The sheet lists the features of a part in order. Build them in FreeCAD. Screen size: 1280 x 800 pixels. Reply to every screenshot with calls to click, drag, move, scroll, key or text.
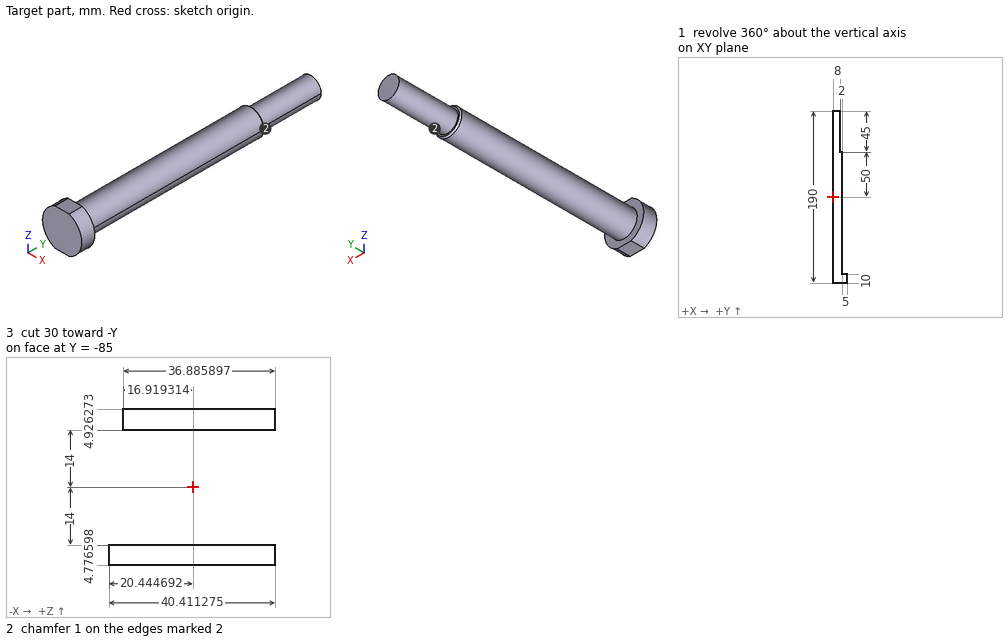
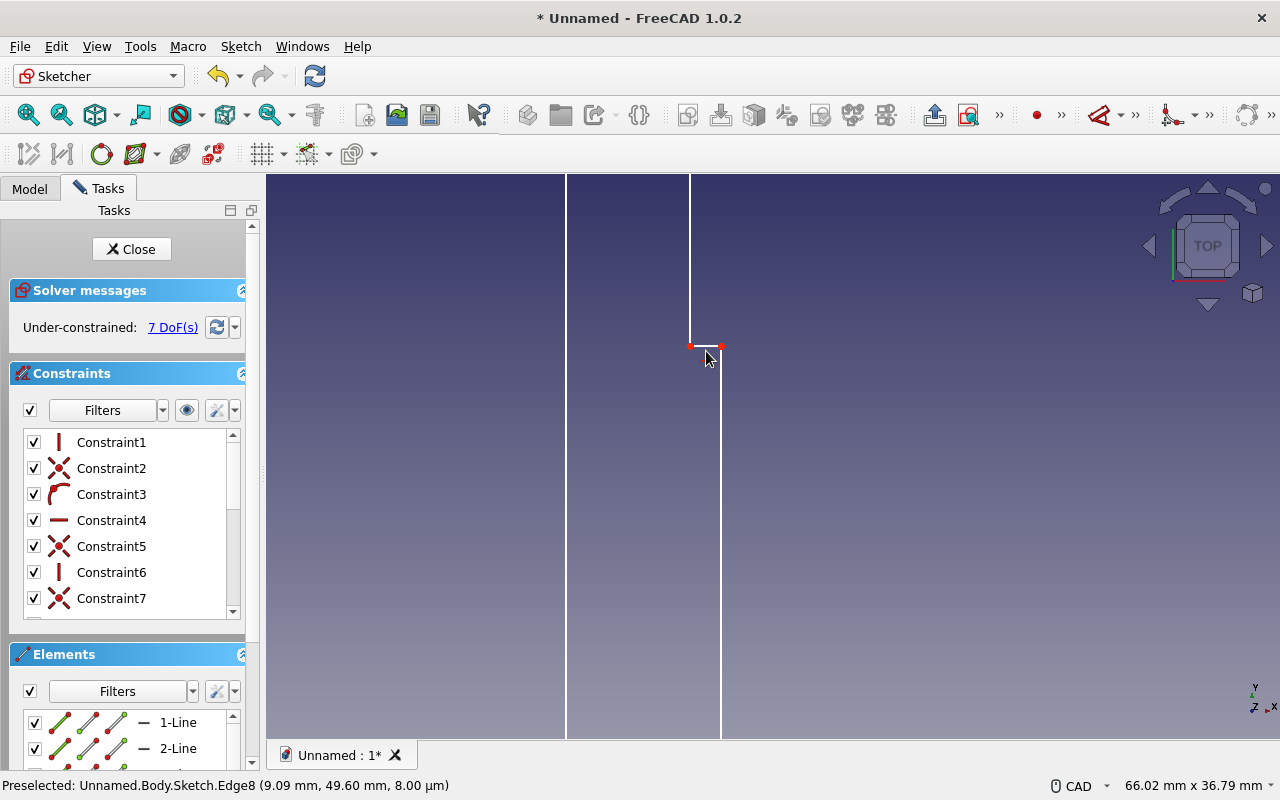
scroll(708, 354, down, 10)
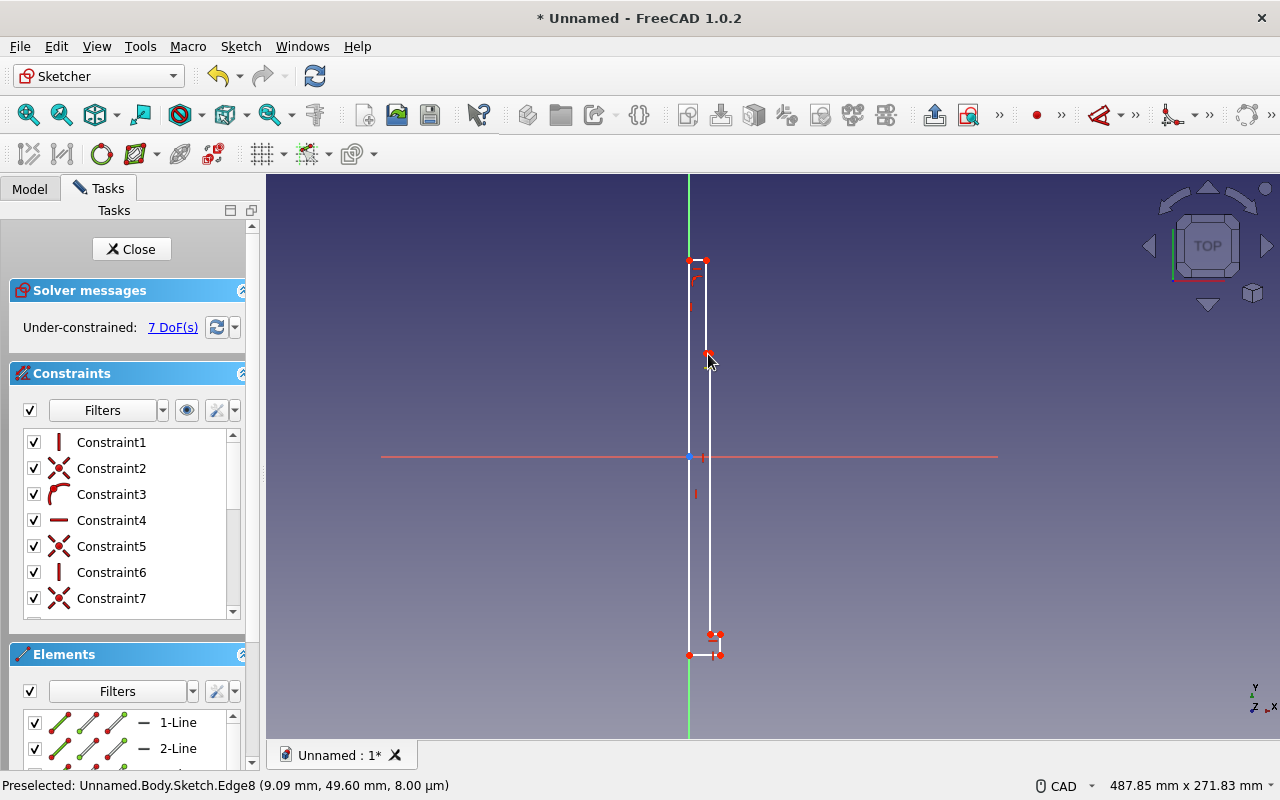
scroll(701, 260, up, 6)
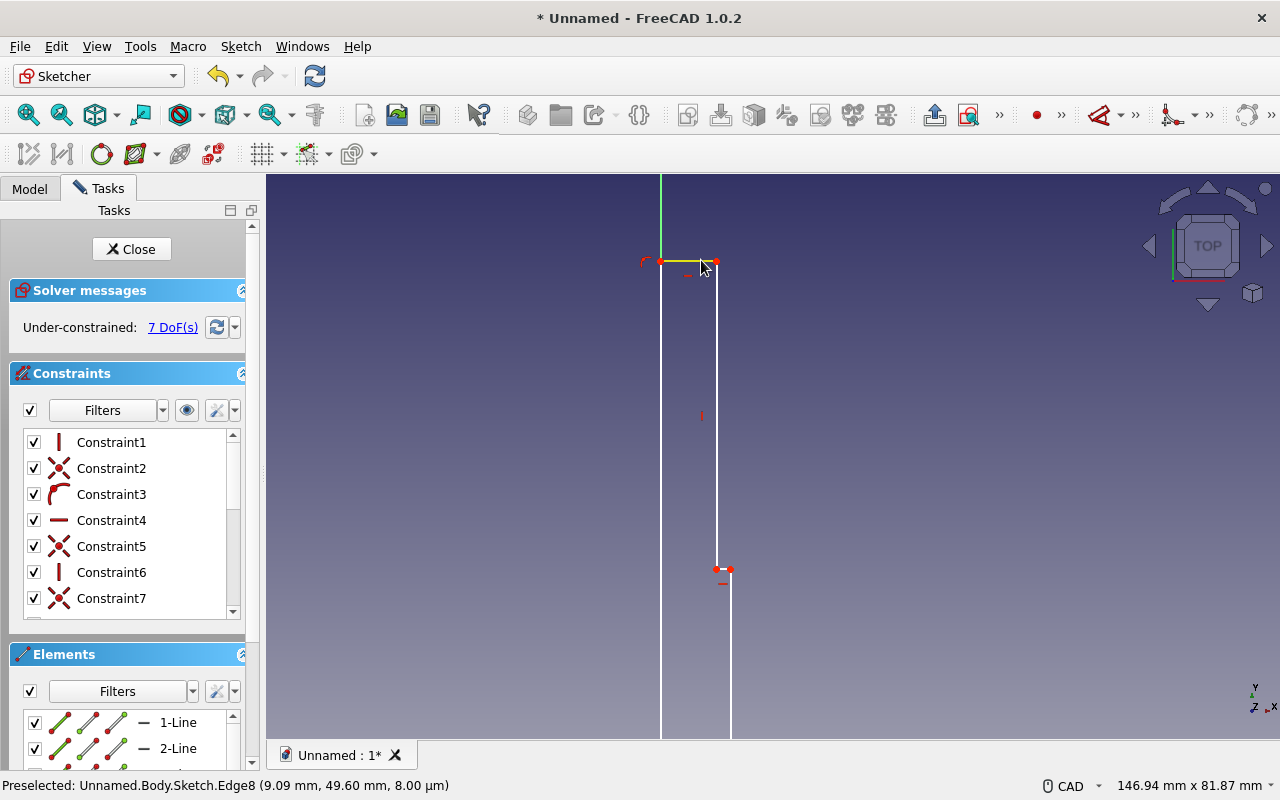
click(700, 261)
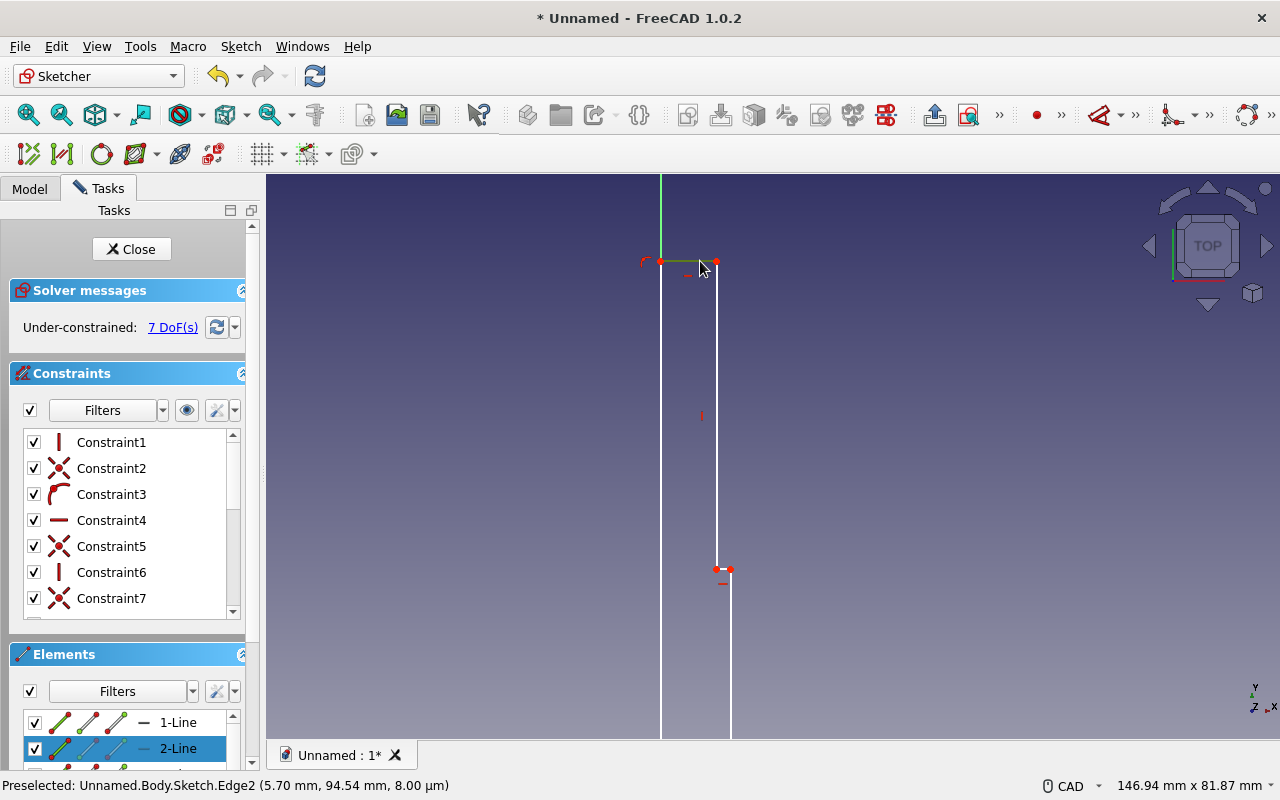
click(1120, 116)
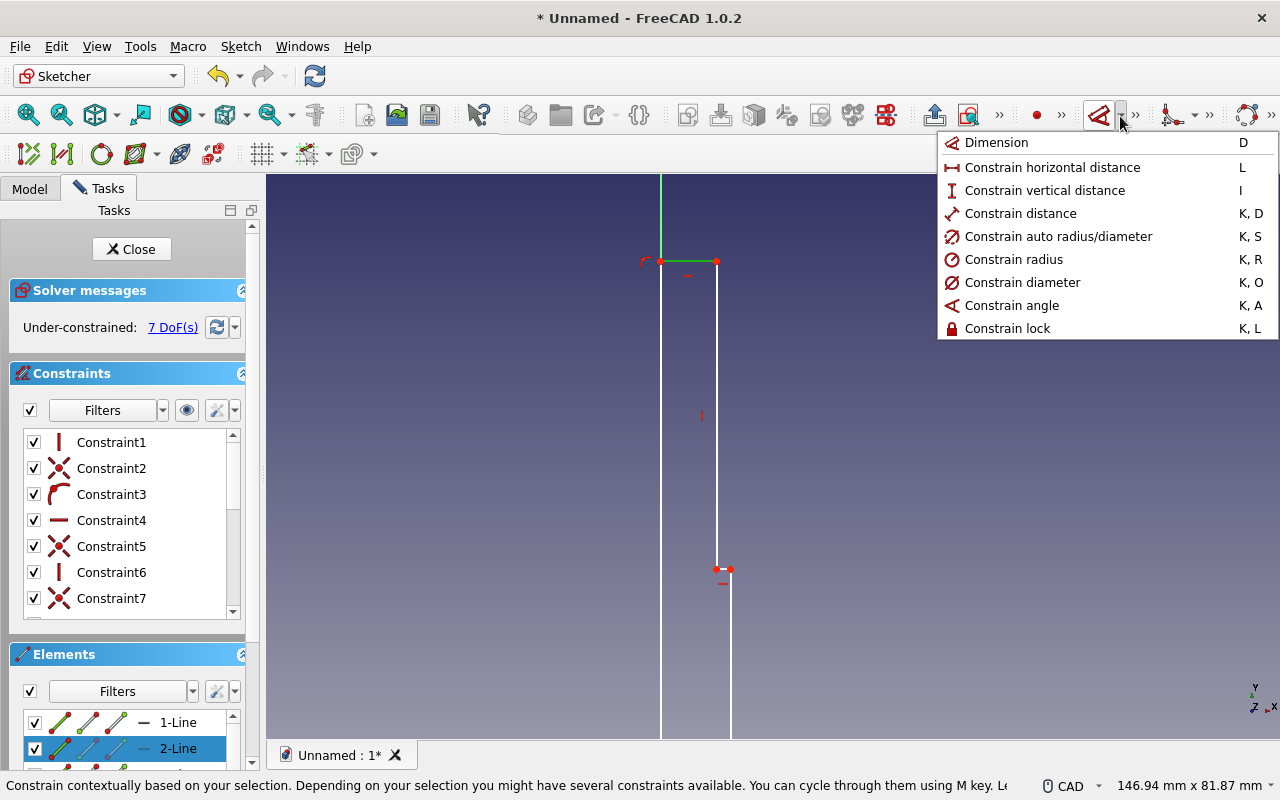
click(1108, 168)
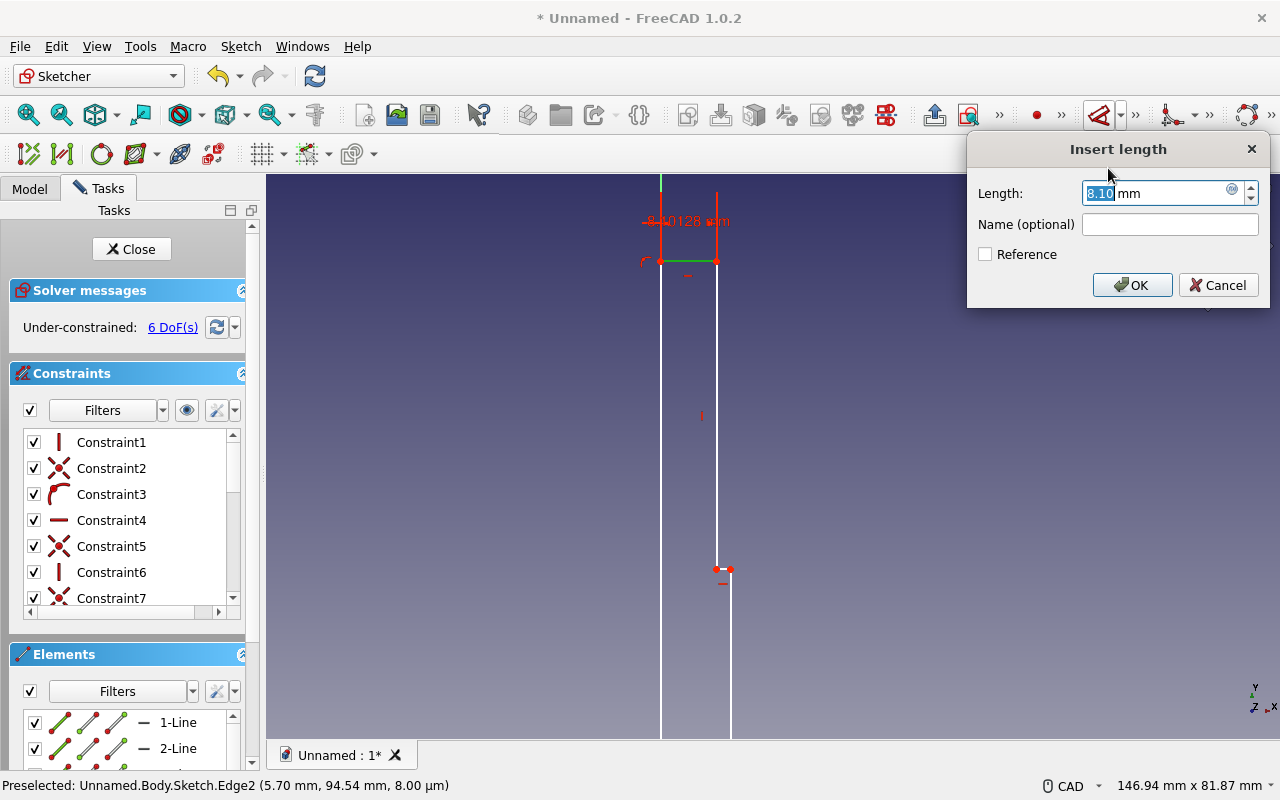
text(8)
key(Return)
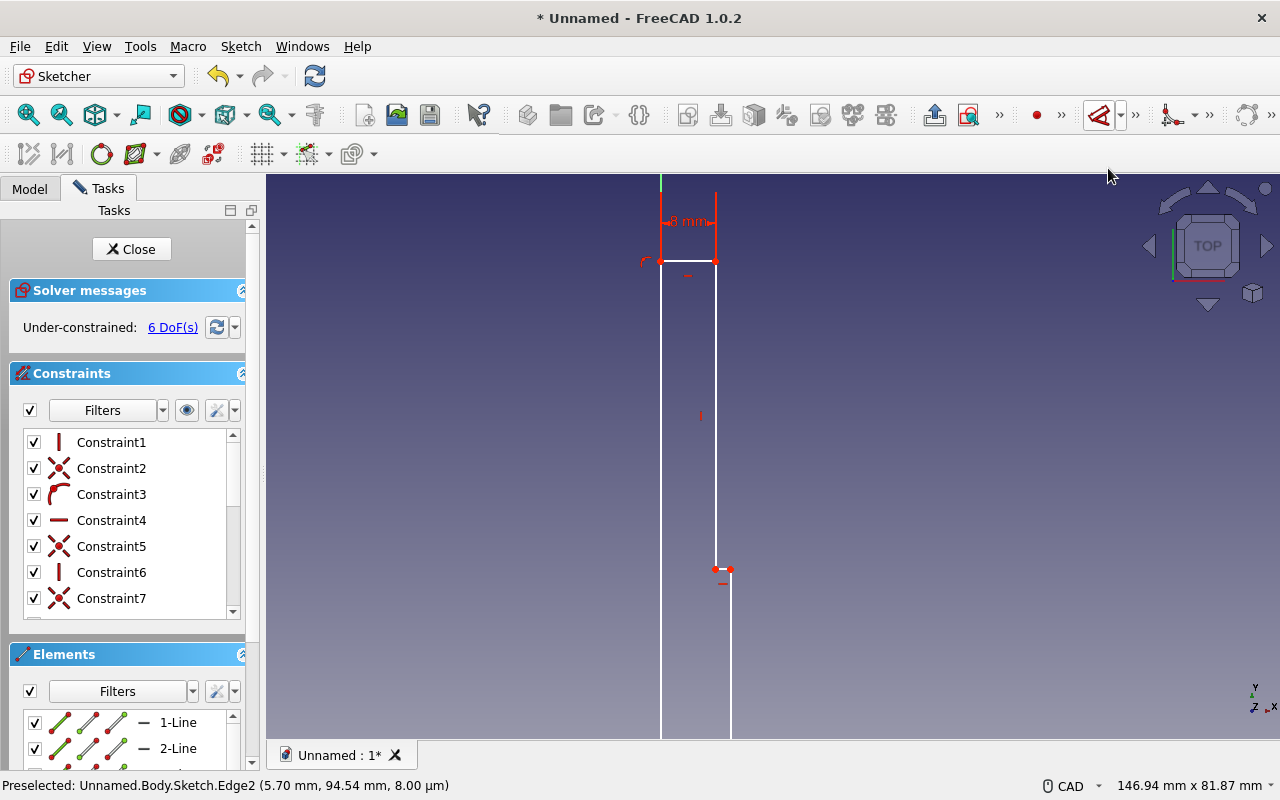
scroll(701, 260, down, 6)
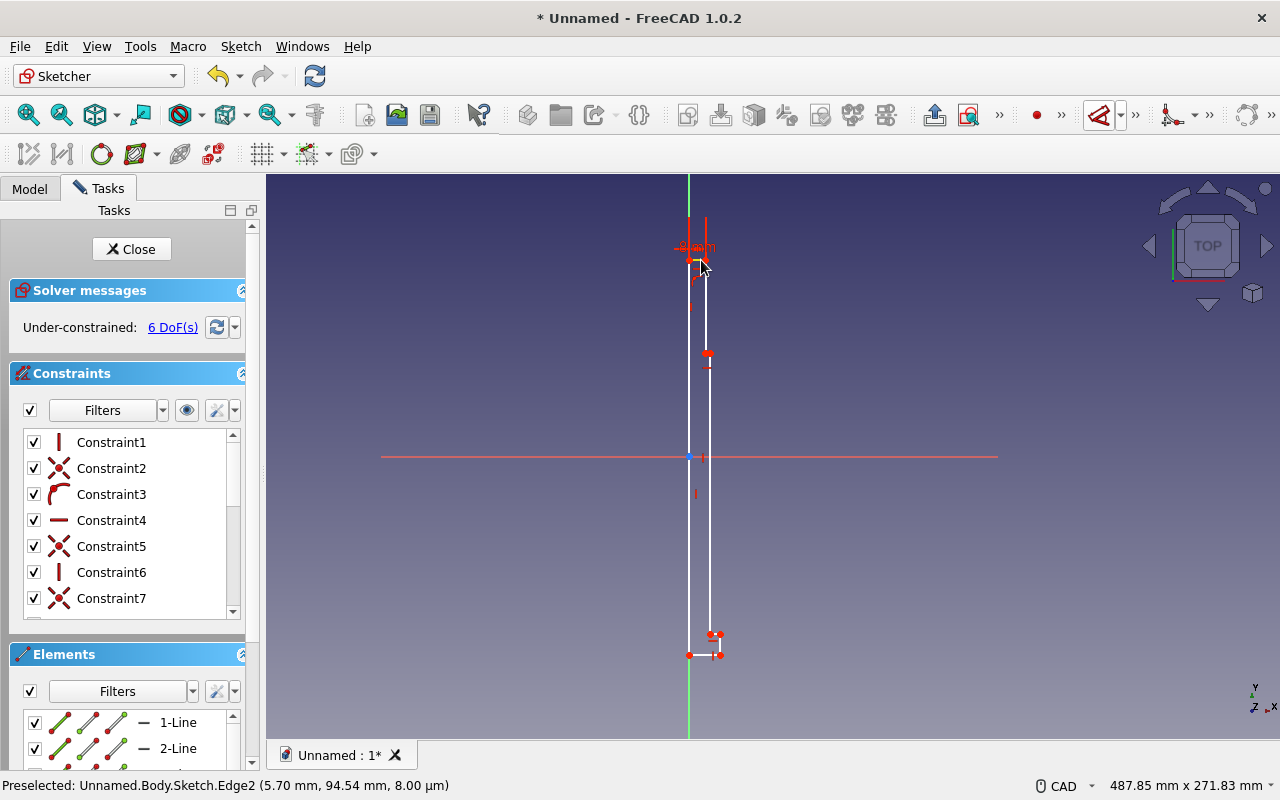
scroll(717, 634, up, 8)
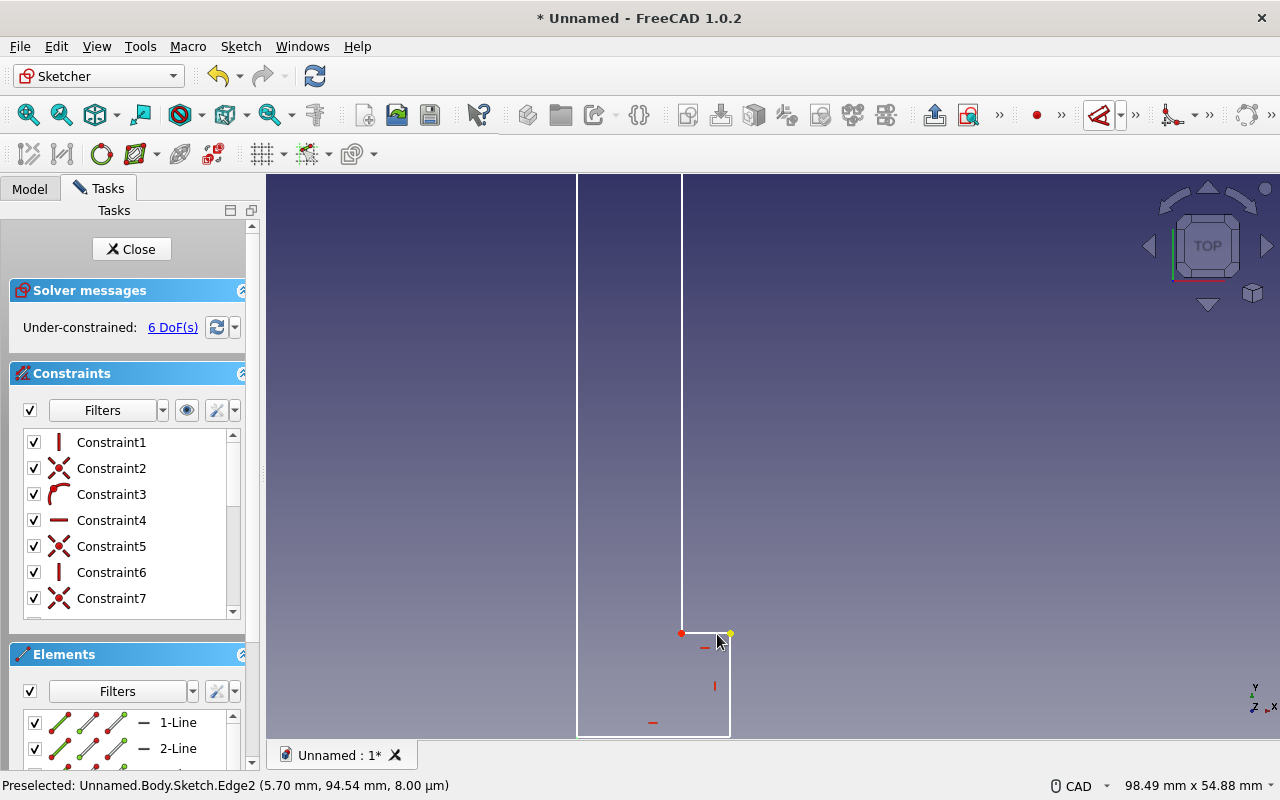
click(716, 633)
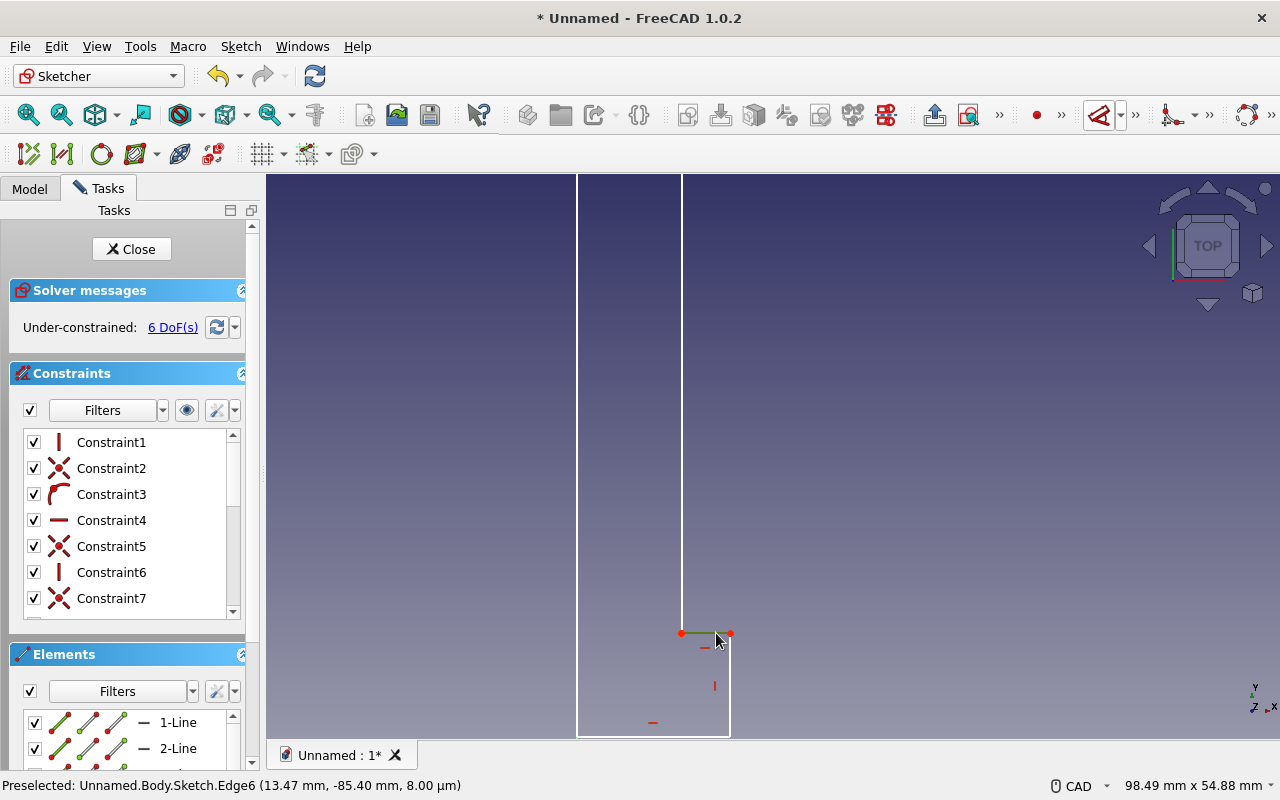
click(1120, 116)